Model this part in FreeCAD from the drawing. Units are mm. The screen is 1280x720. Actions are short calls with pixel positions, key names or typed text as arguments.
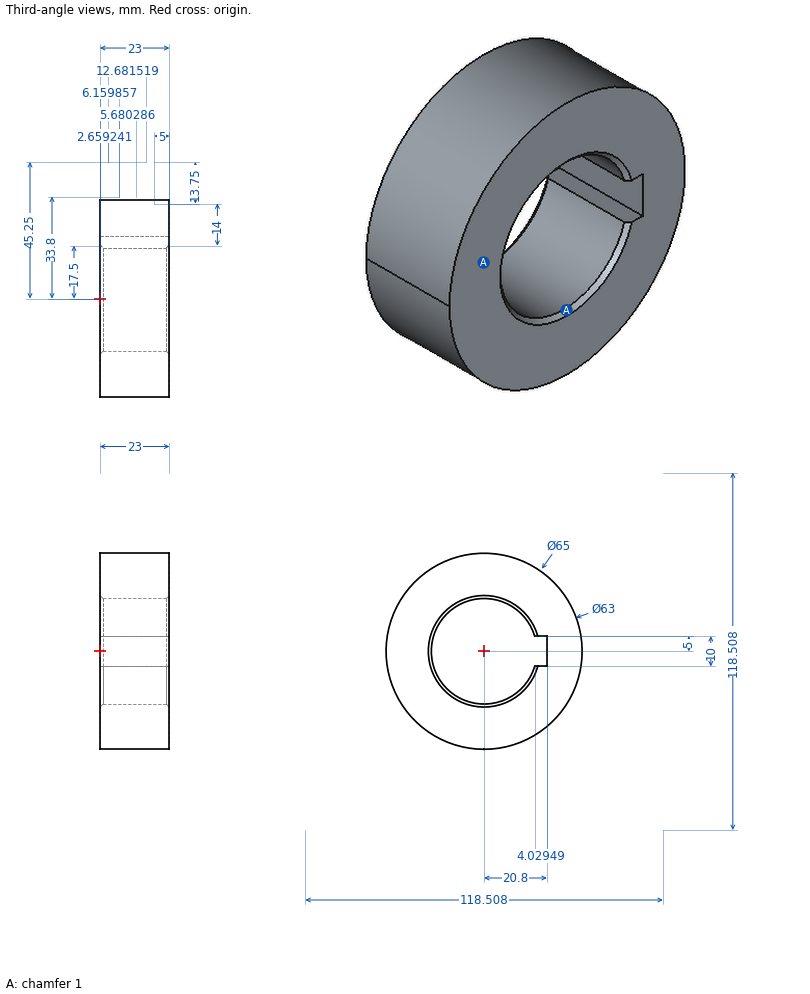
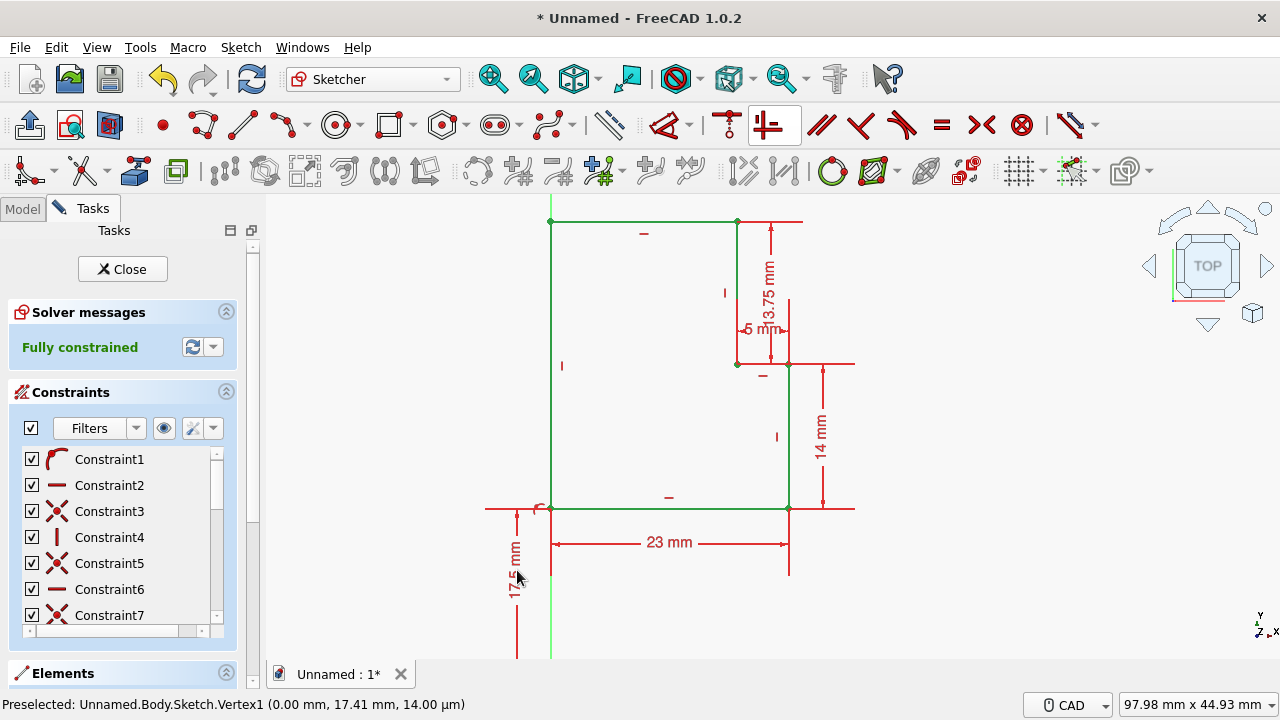
click(123, 269)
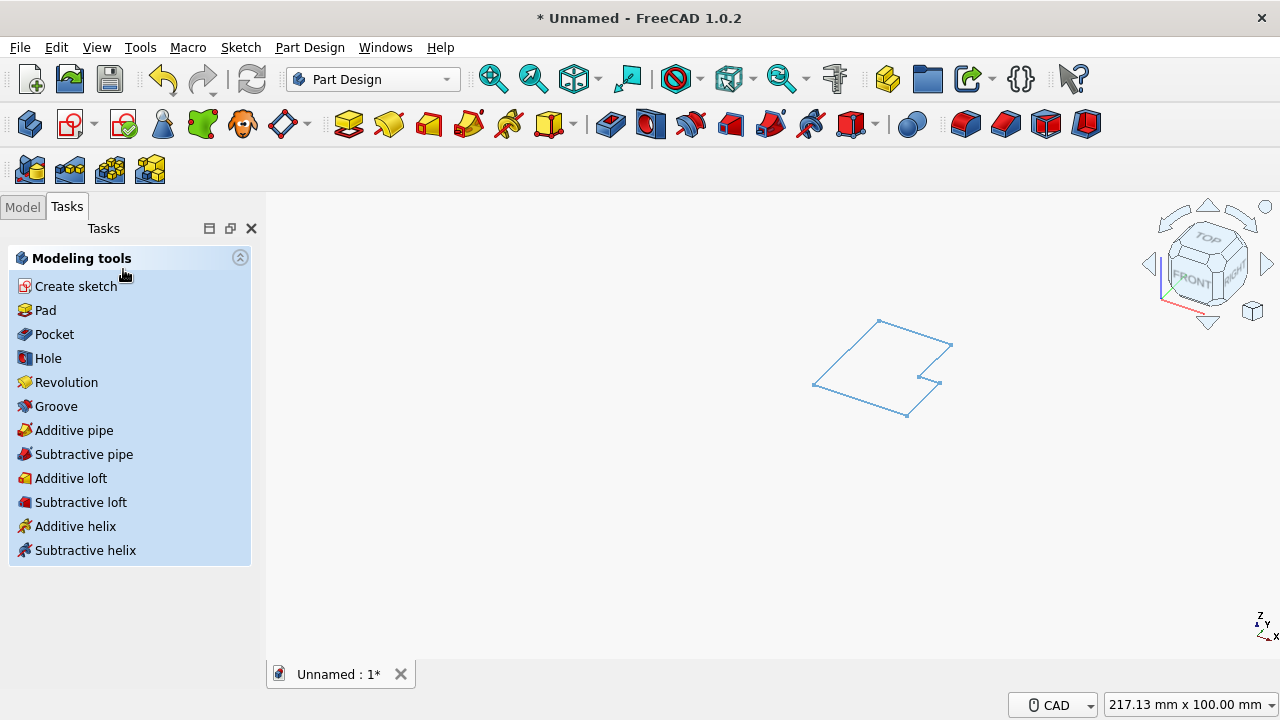
click(390, 124)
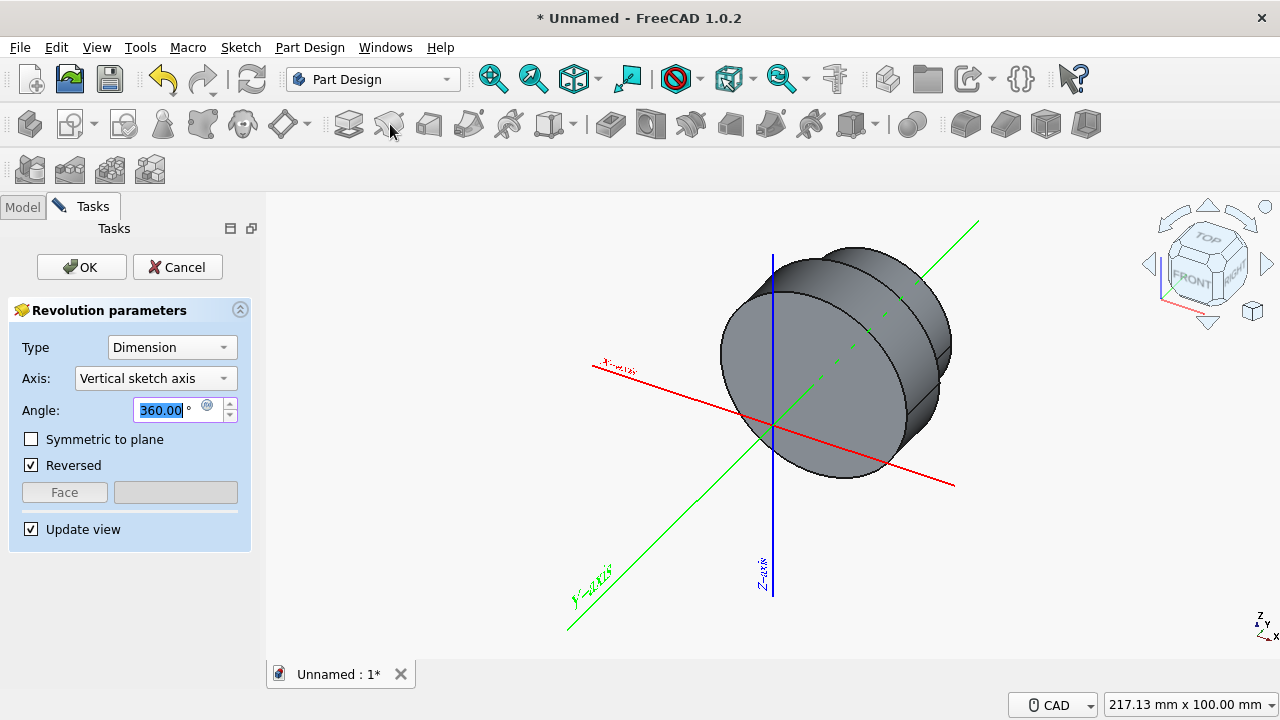
click(156, 378)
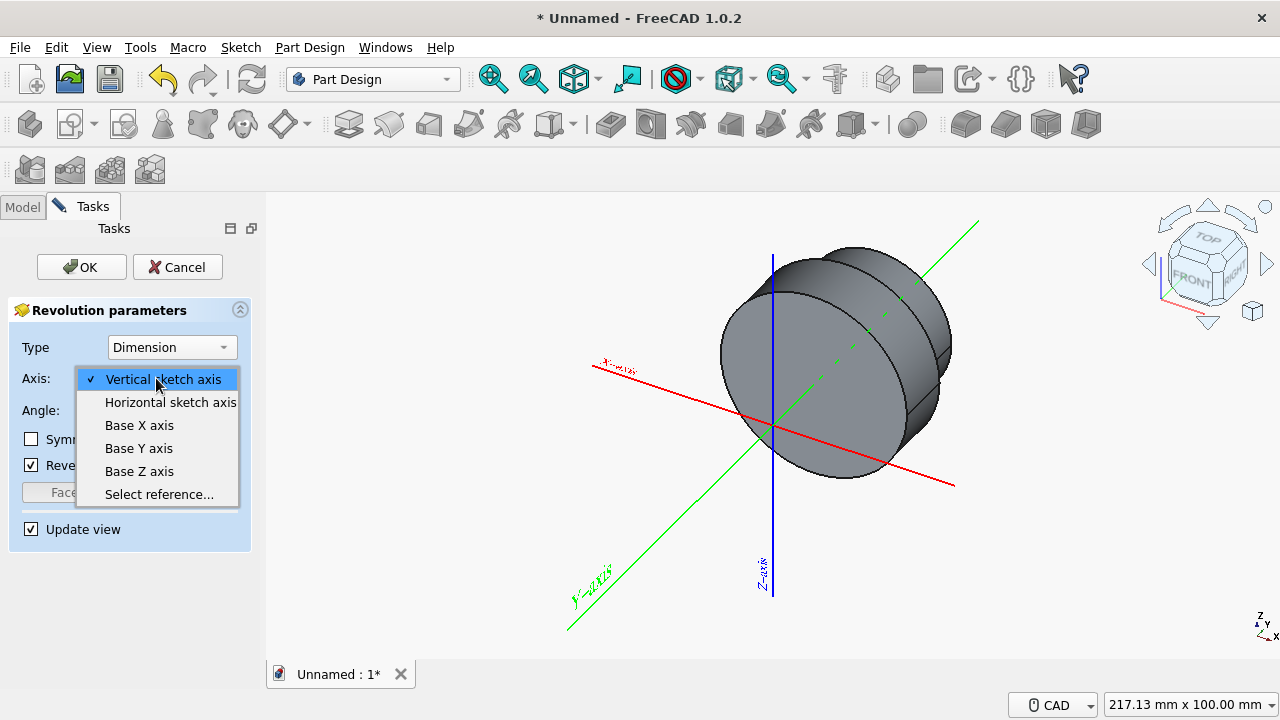
click(156, 402)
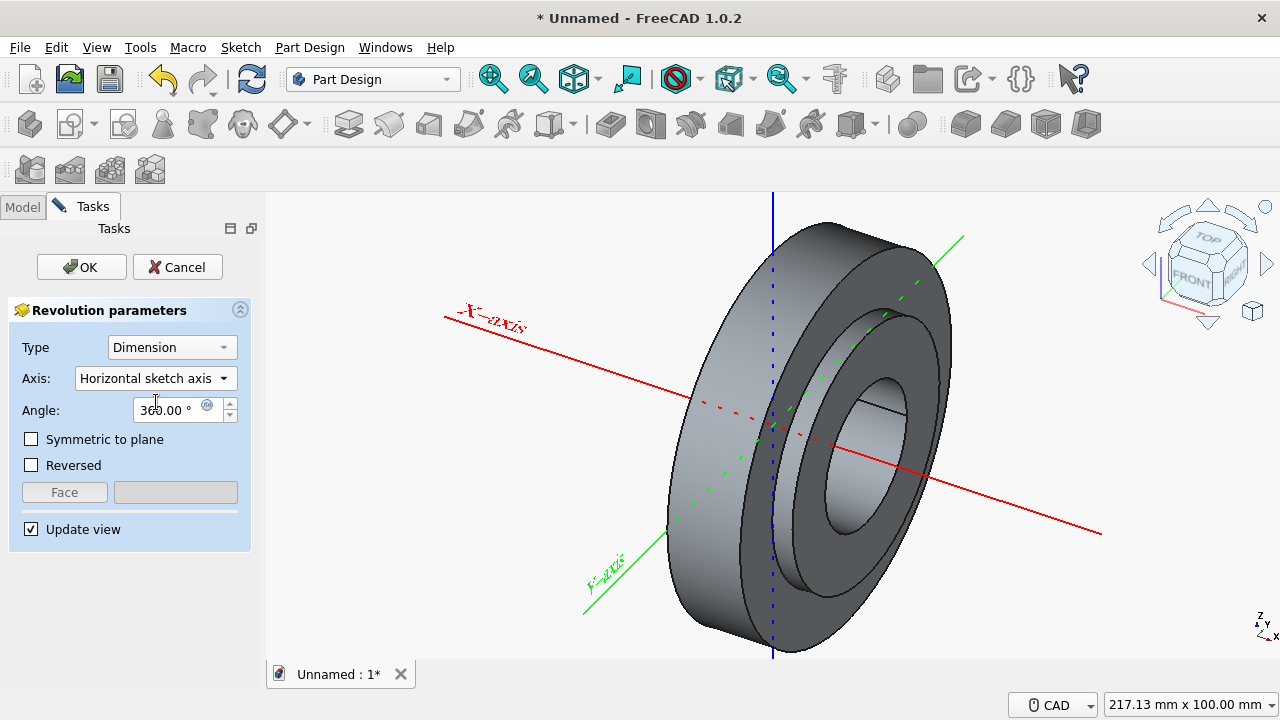
click(82, 267)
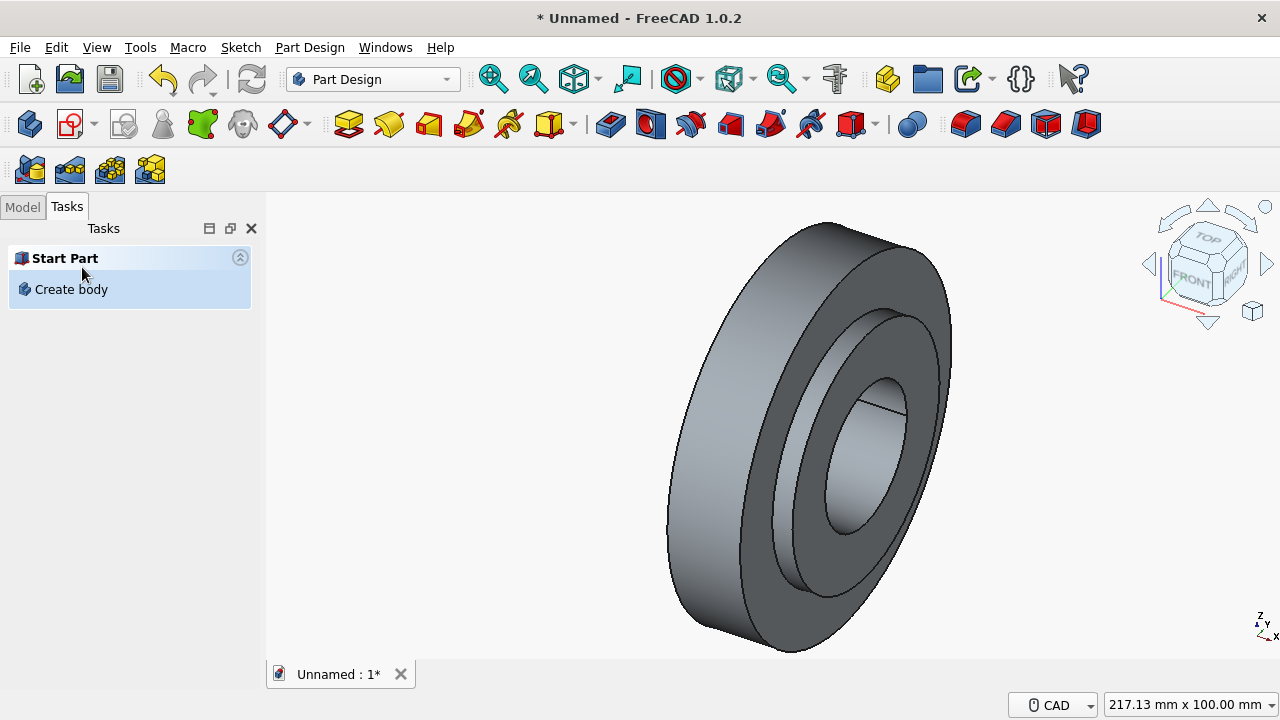
key(v)
key(f)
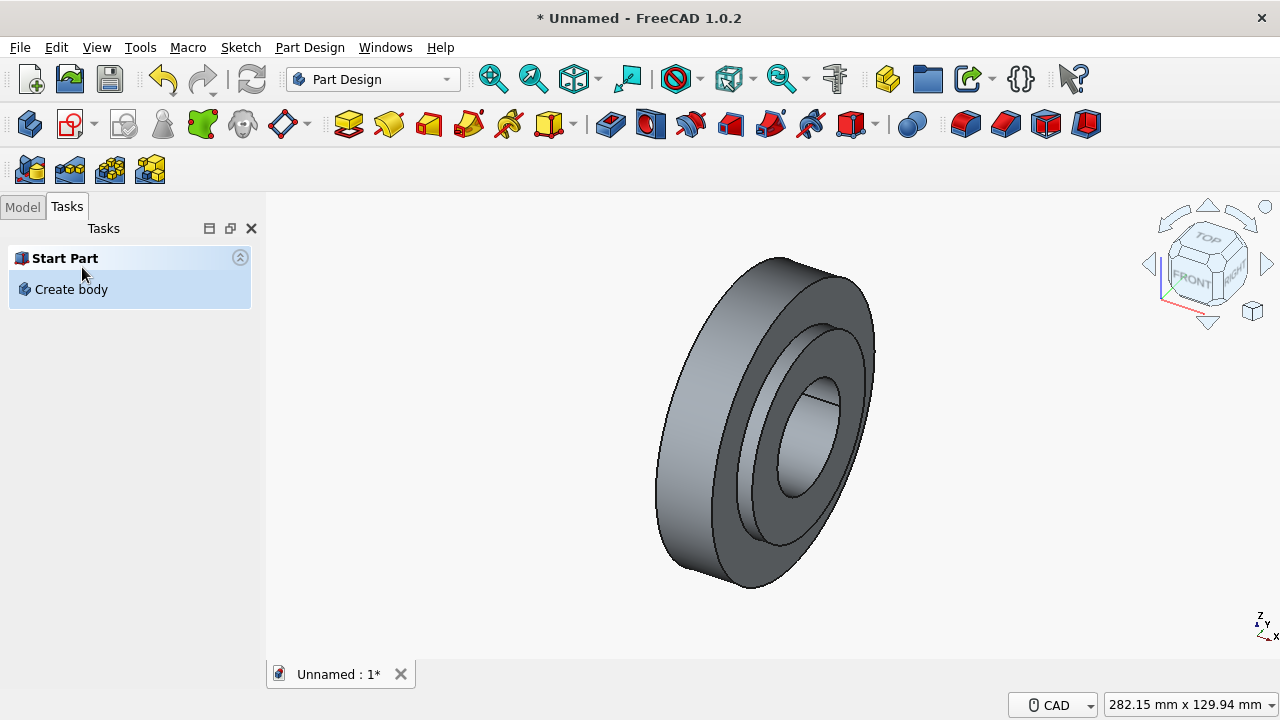
click(70, 124)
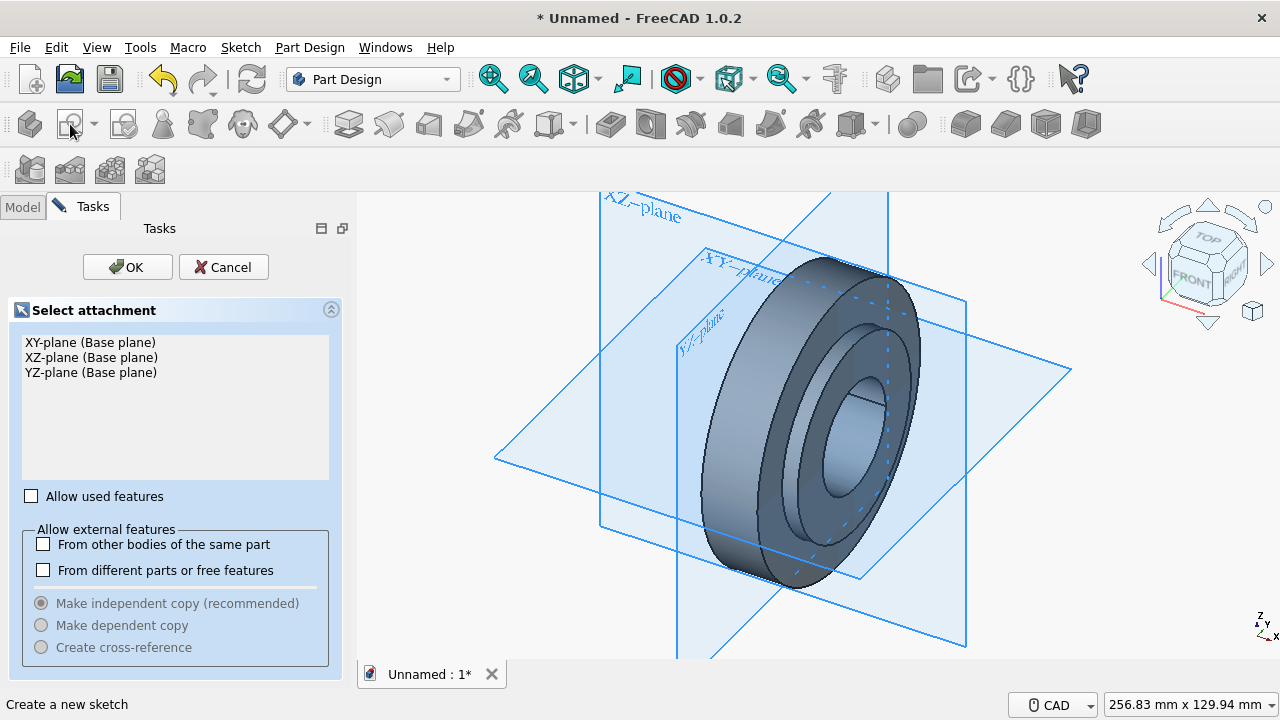
click(82, 342)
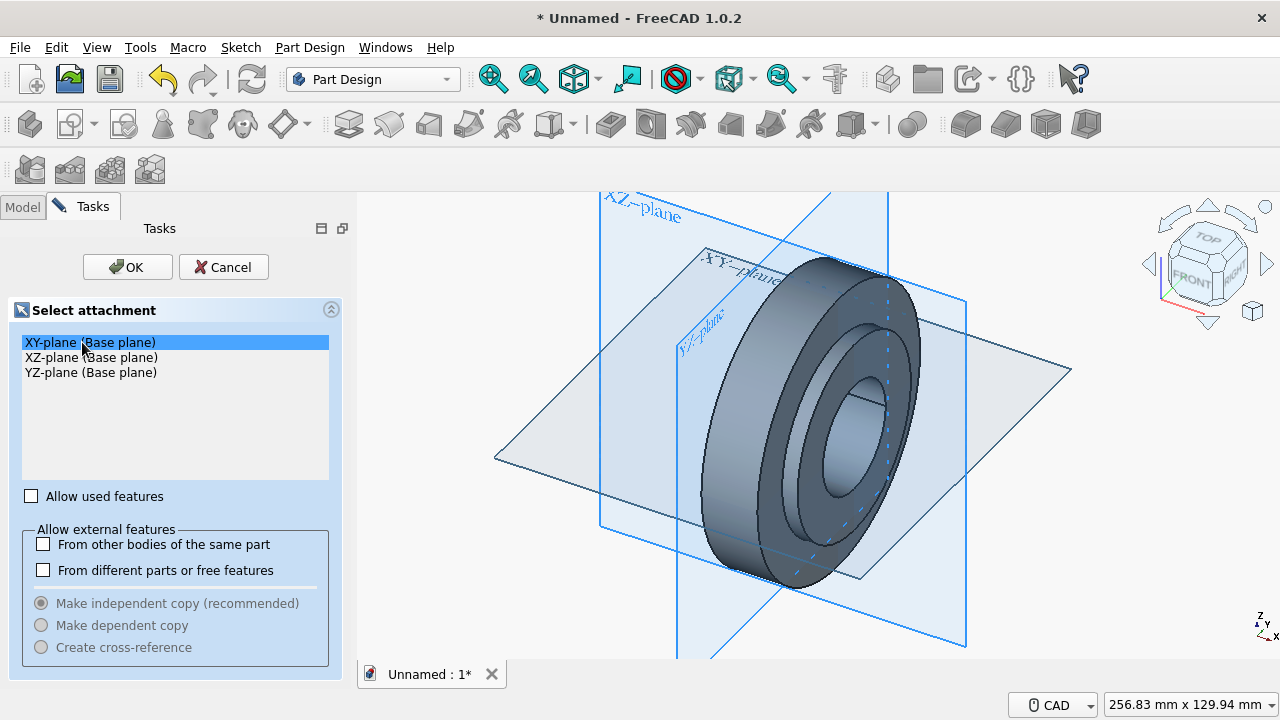
click(128, 267)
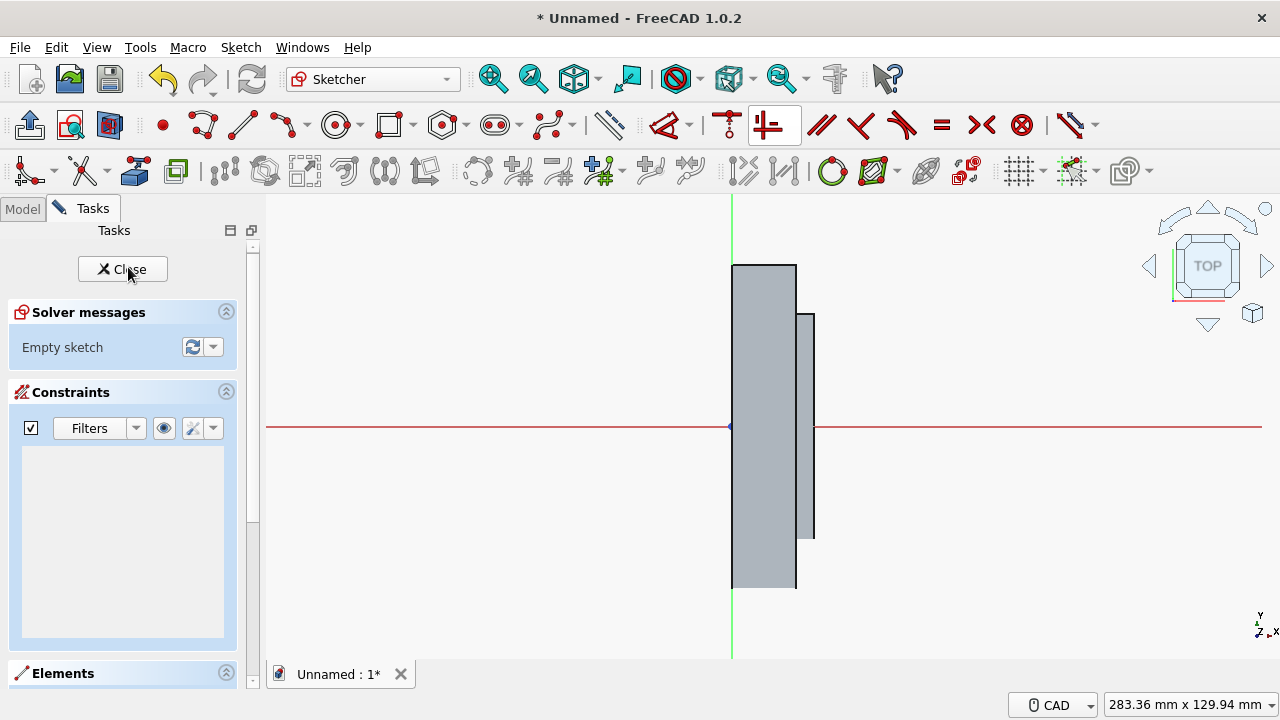
key(q)
key(s)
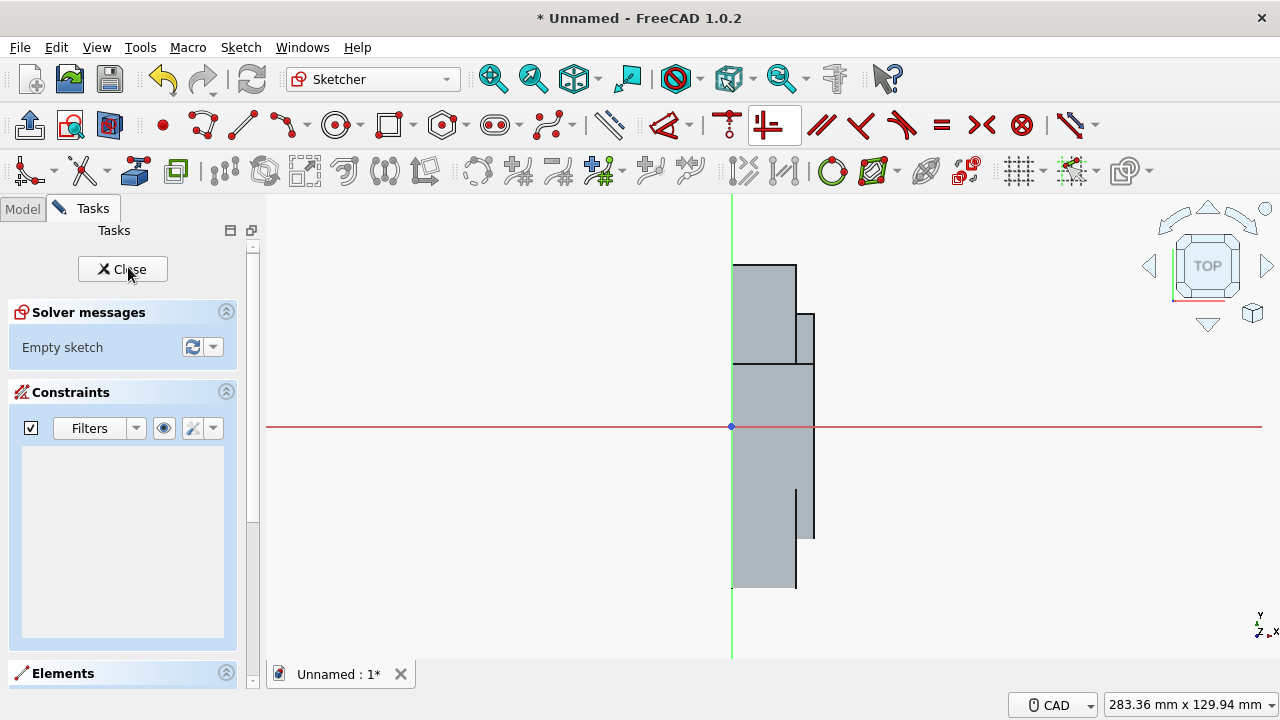
scroll(773, 263, up, 10)